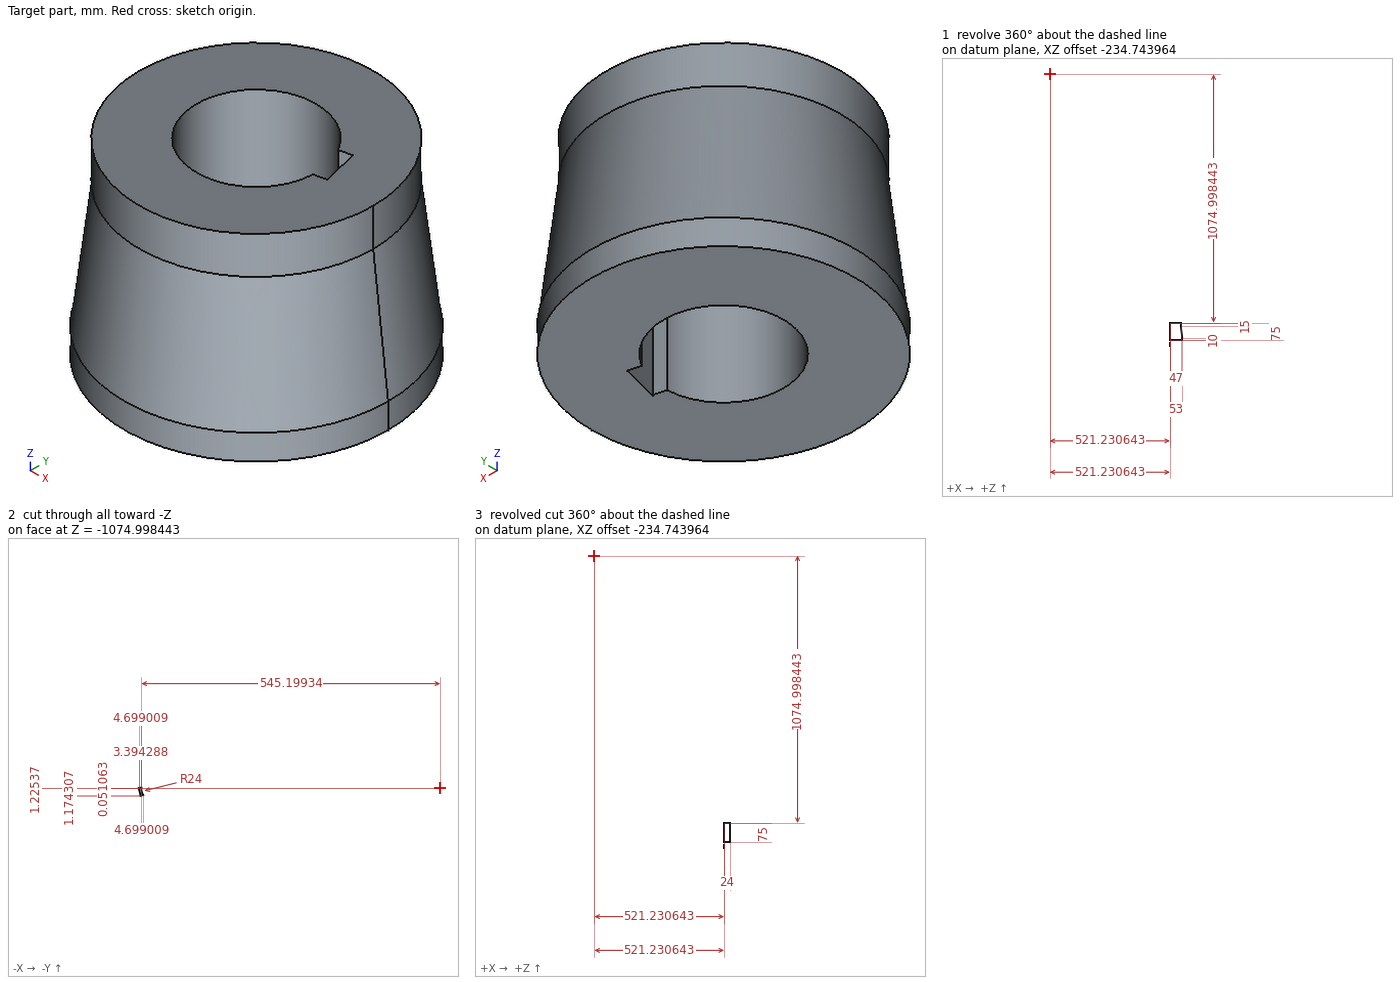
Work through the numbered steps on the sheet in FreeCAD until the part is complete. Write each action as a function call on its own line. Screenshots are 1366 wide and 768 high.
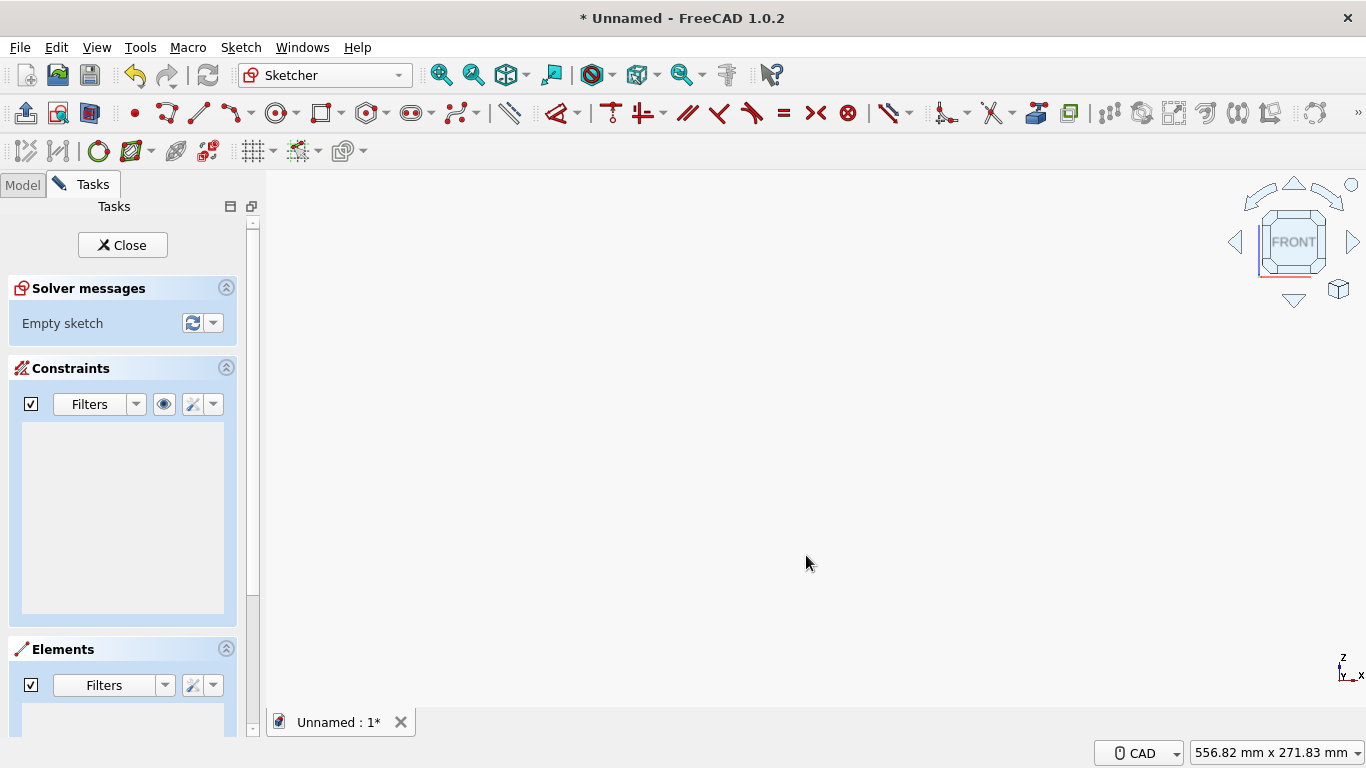
click(168, 114)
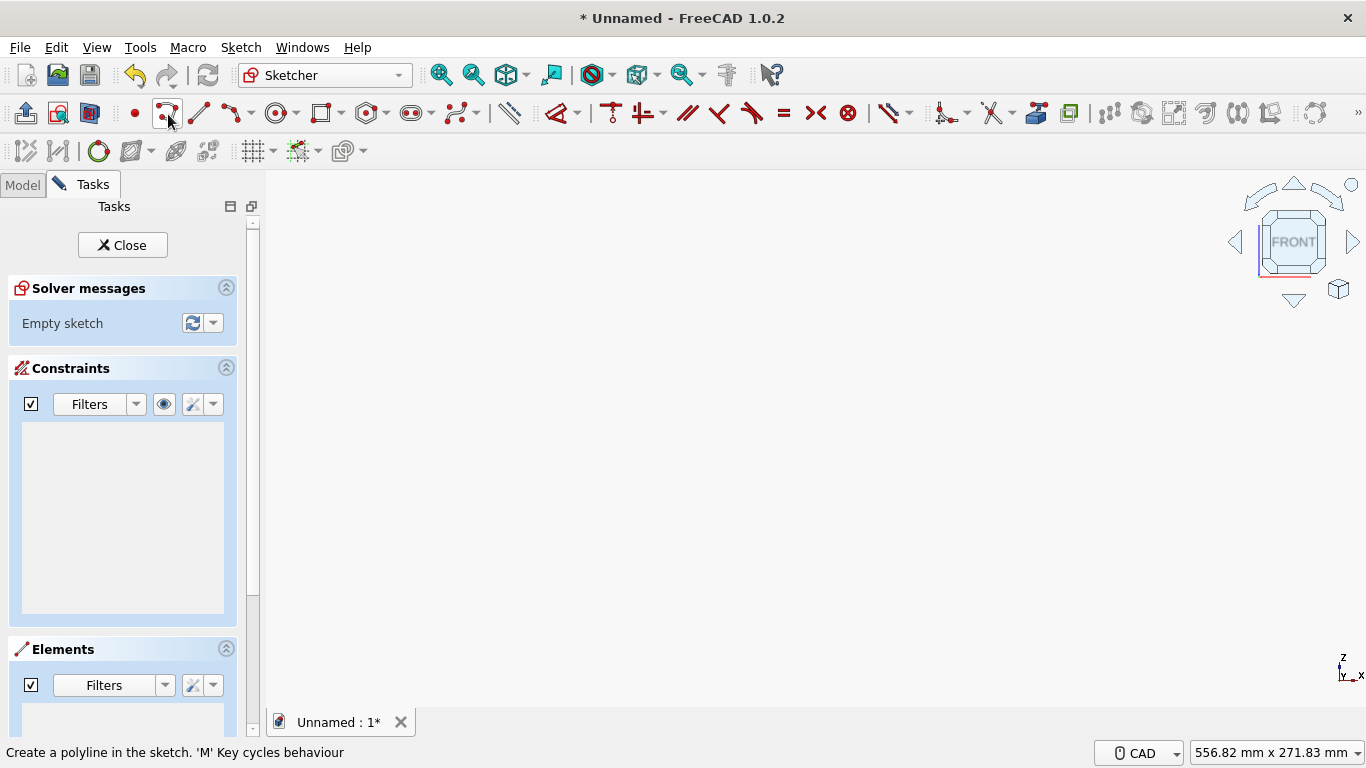
click(695, 325)
click(695, 473)
click(800, 473)
click(800, 453)
click(788, 355)
click(788, 325)
click(695, 326)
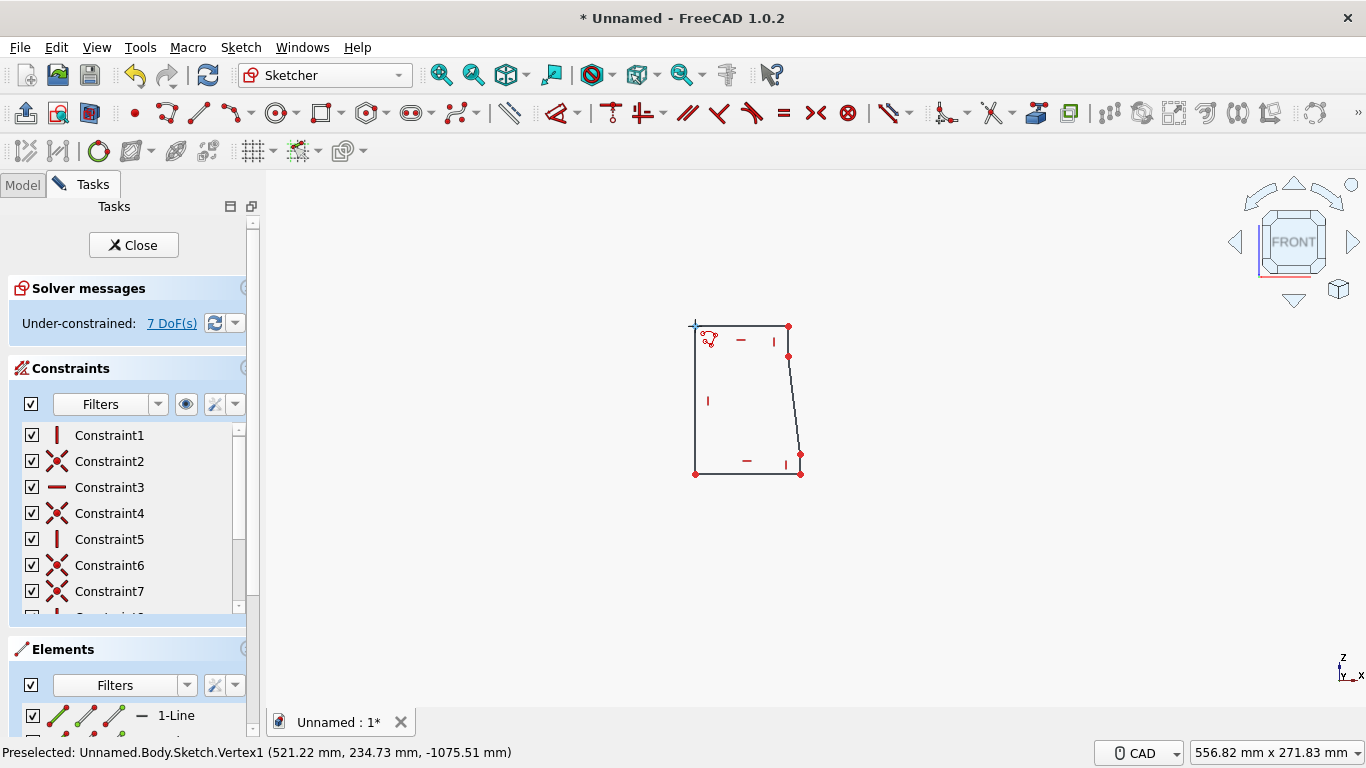
click(200, 114)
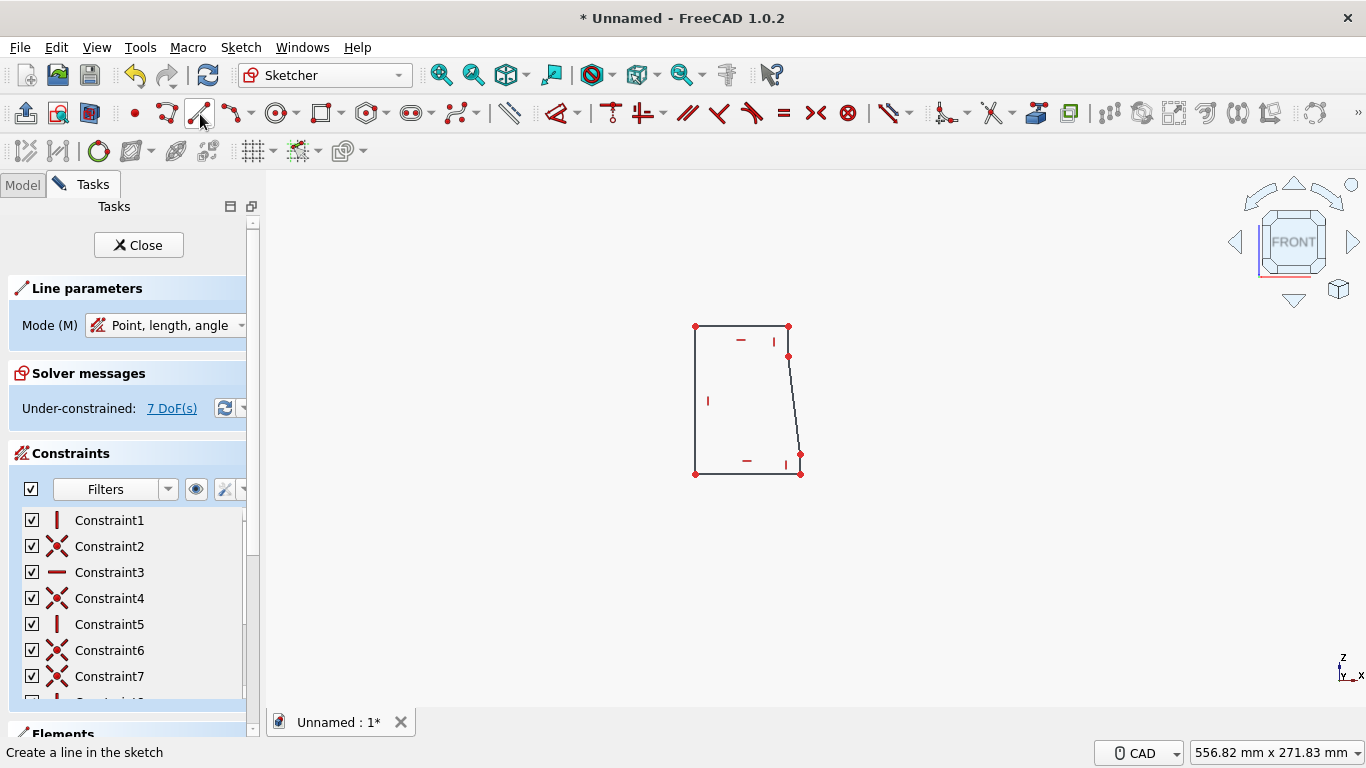
click(695, 488)
click(695, 532)
key(Escape)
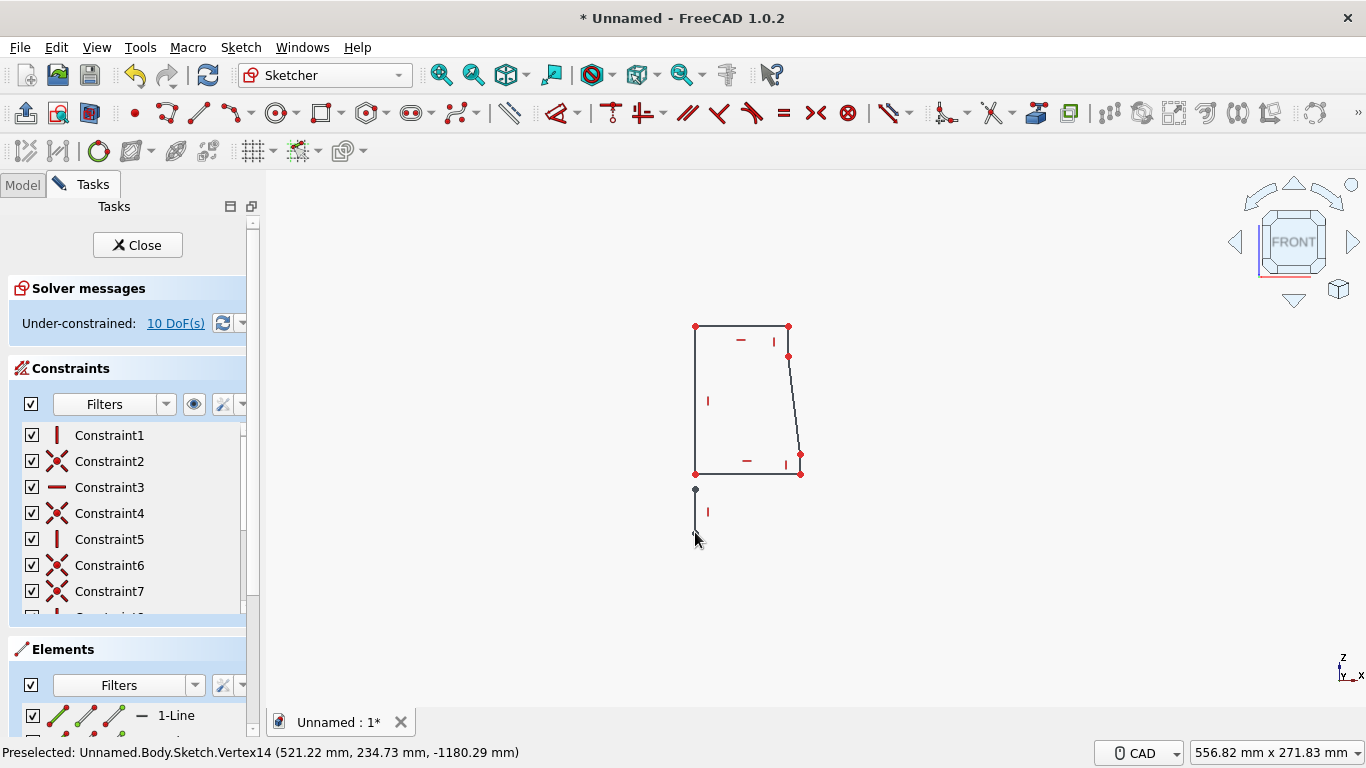
click(695, 502)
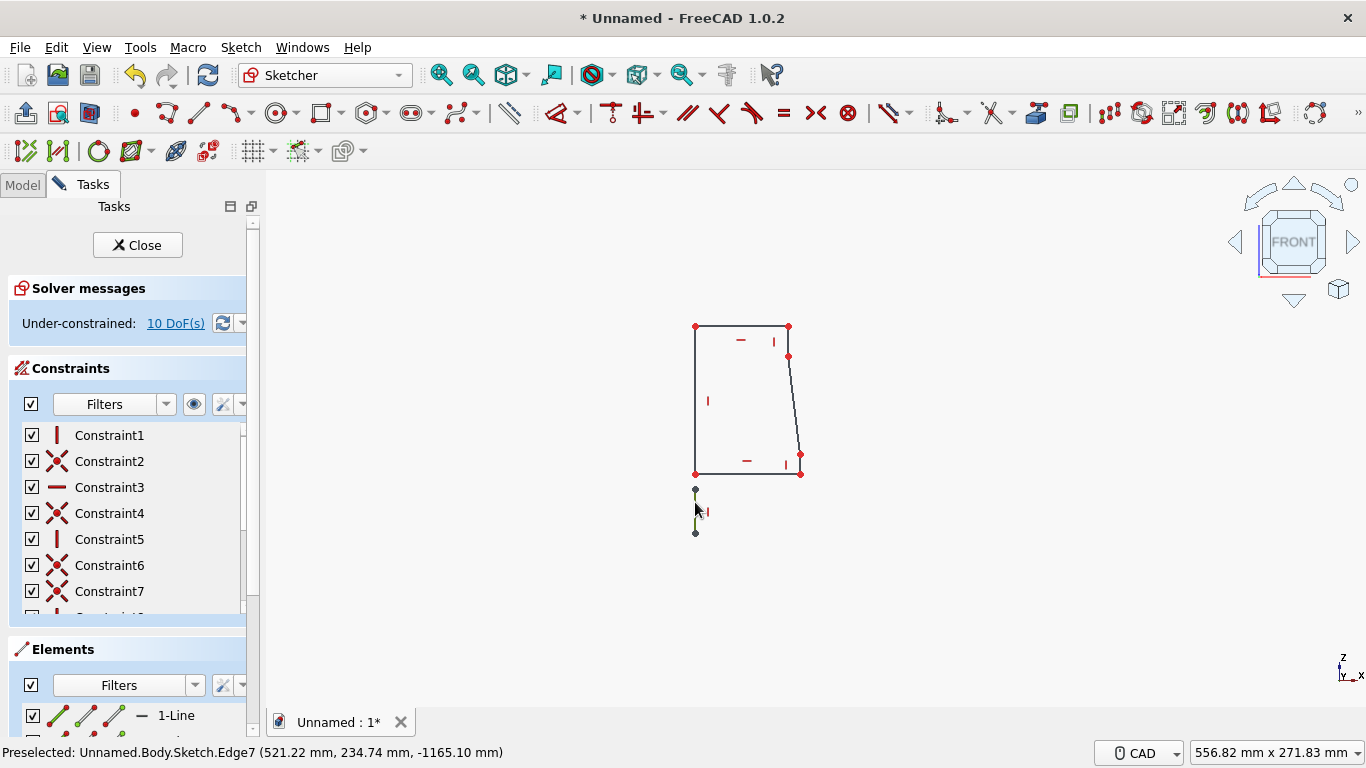
click(510, 114)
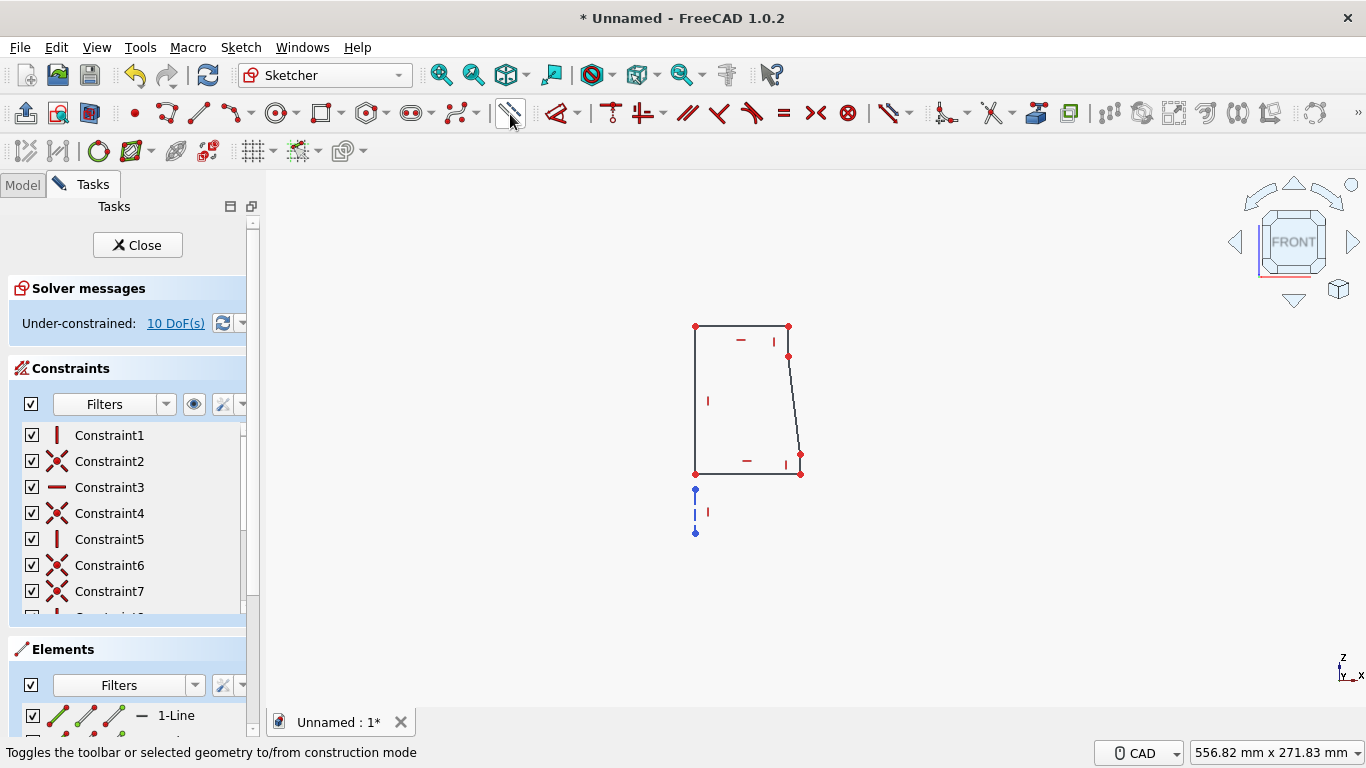
click(556, 114)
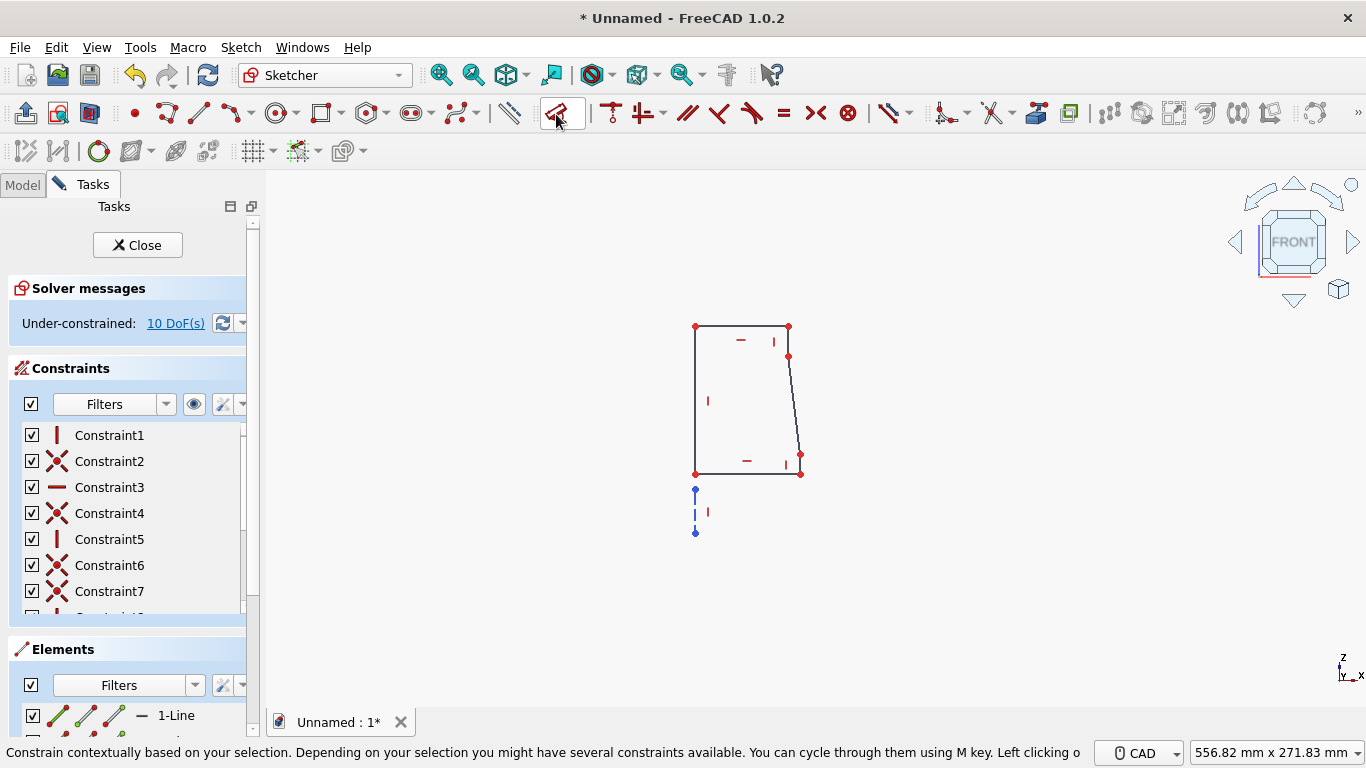
click(695, 370)
click(661, 400)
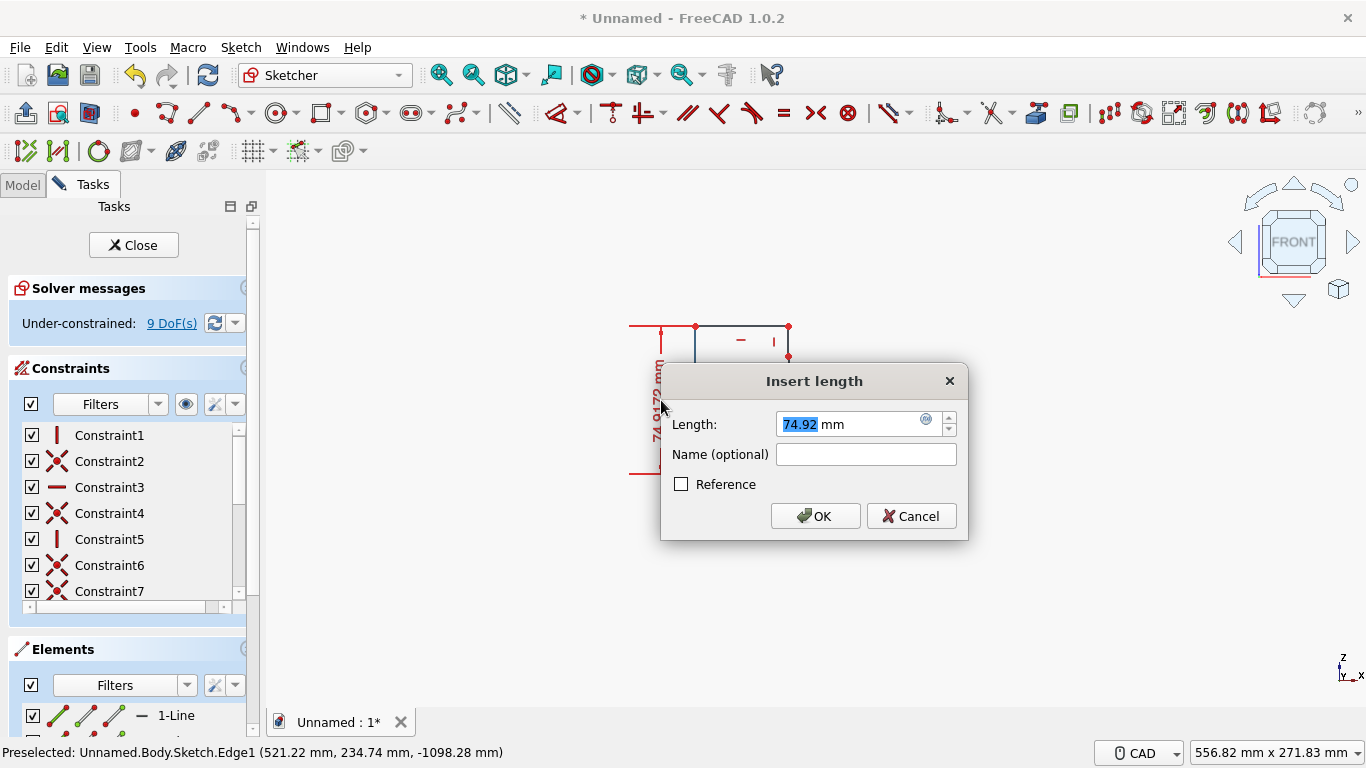
text(75)
key(Return)